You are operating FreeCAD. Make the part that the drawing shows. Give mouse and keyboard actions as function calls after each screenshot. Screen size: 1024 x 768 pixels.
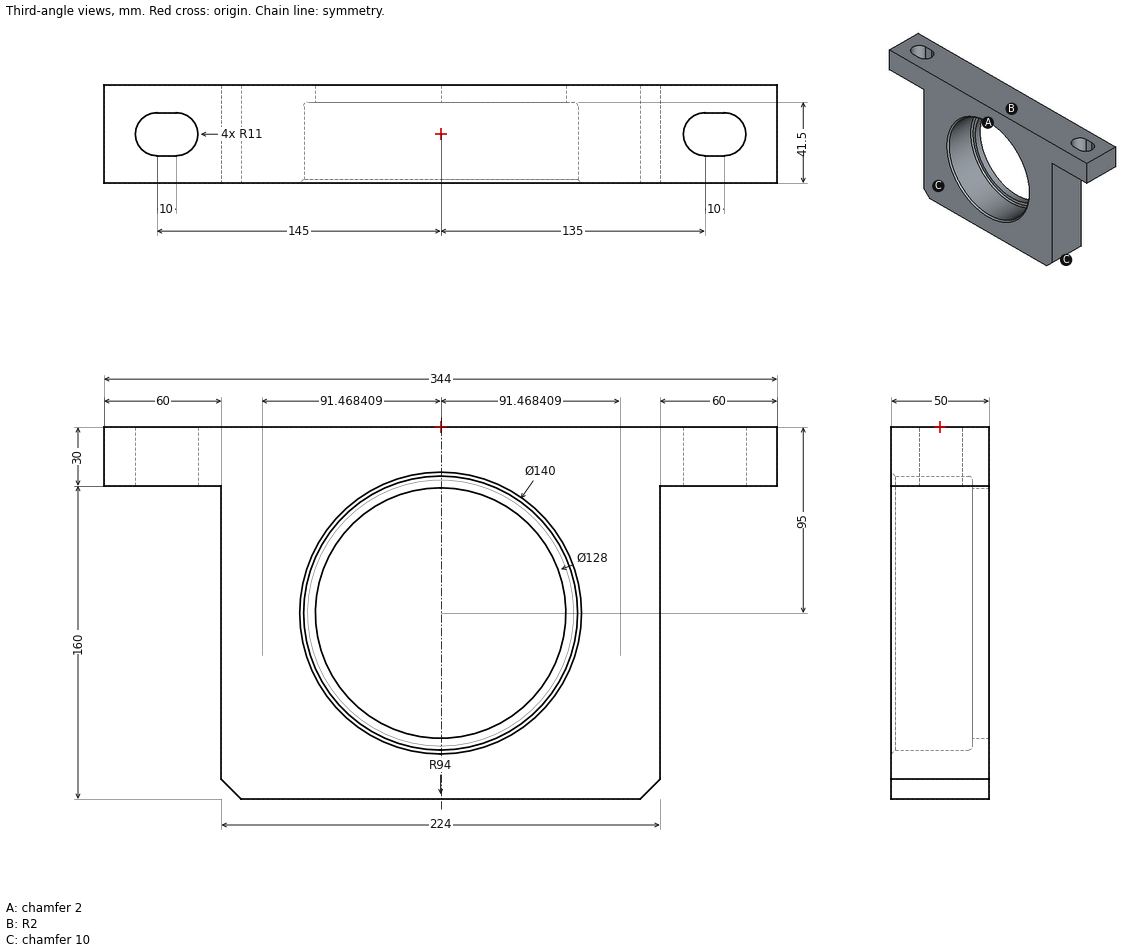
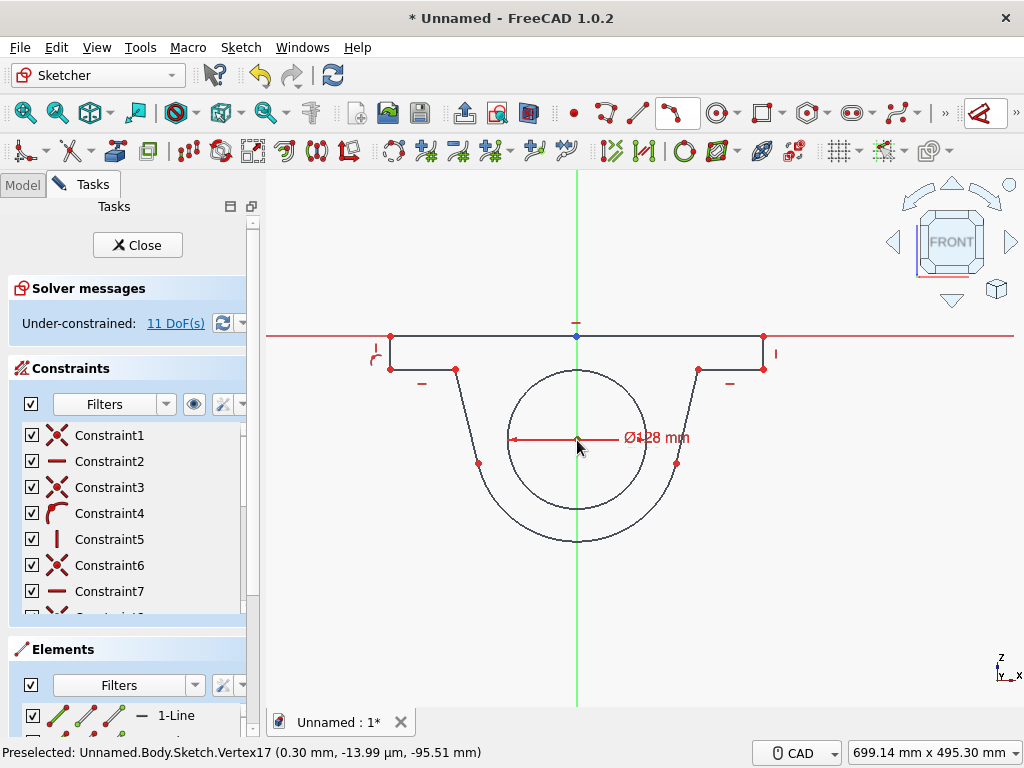
click(577, 645)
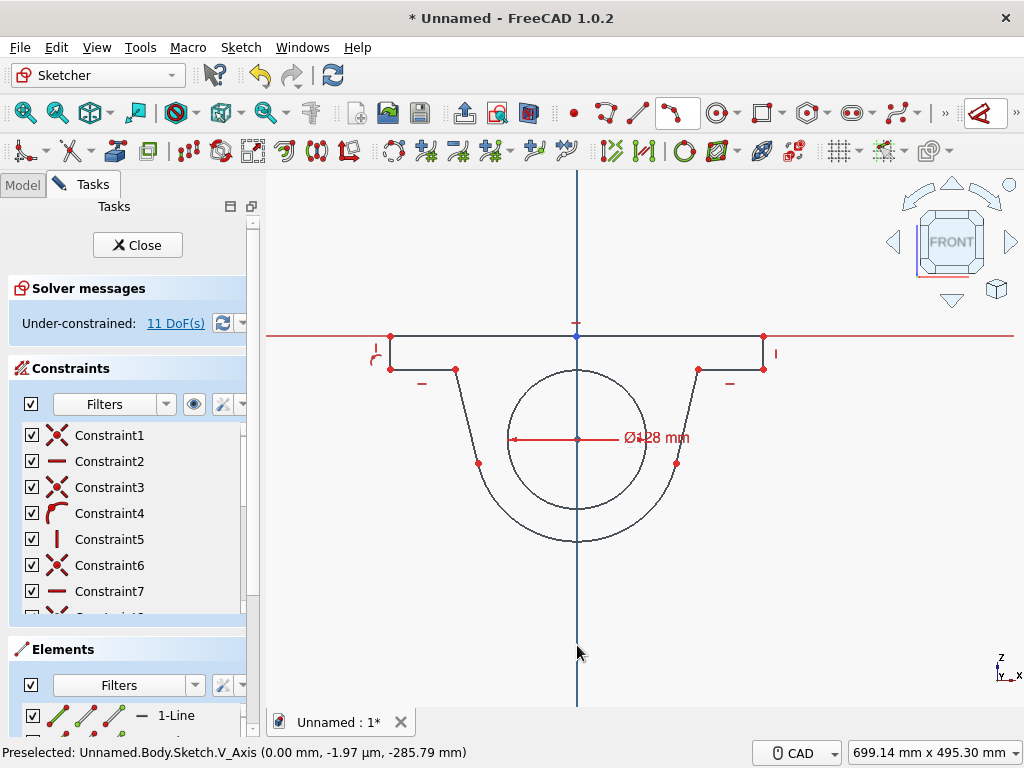
key(c)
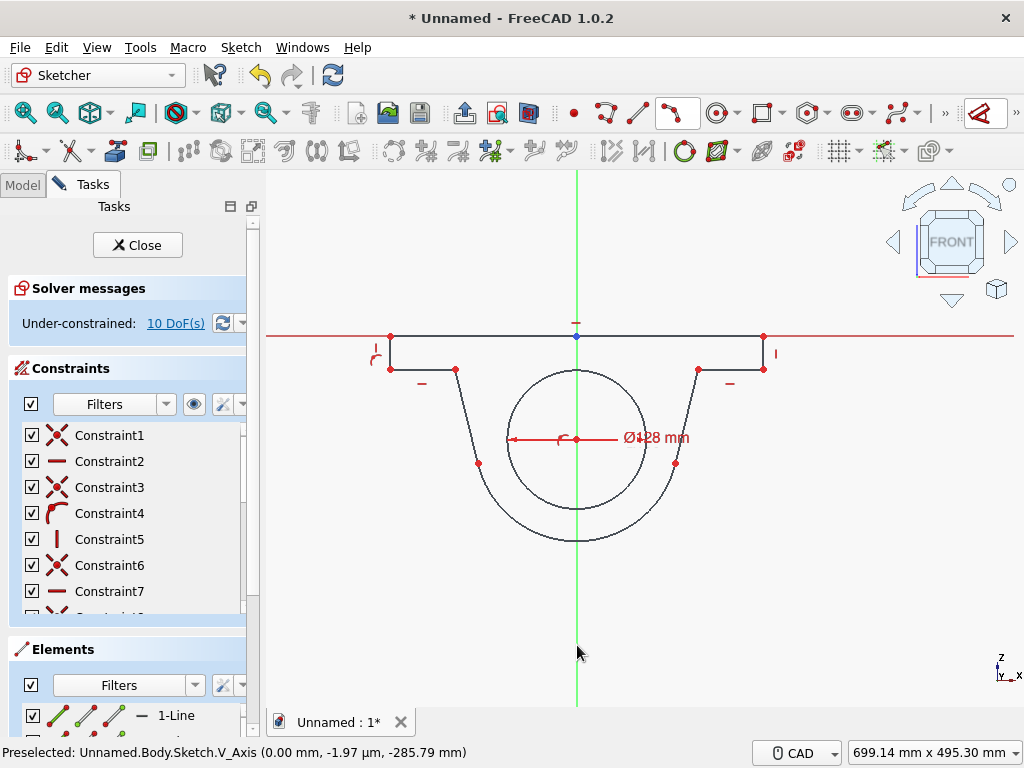
click(390, 370)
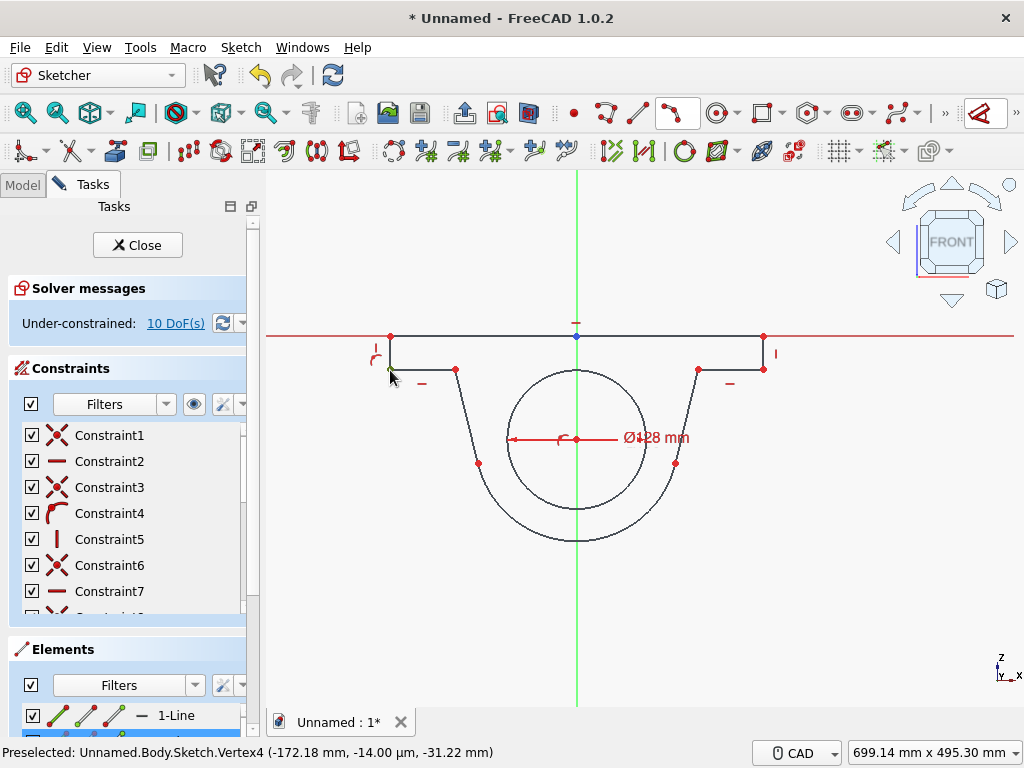
click(763, 370)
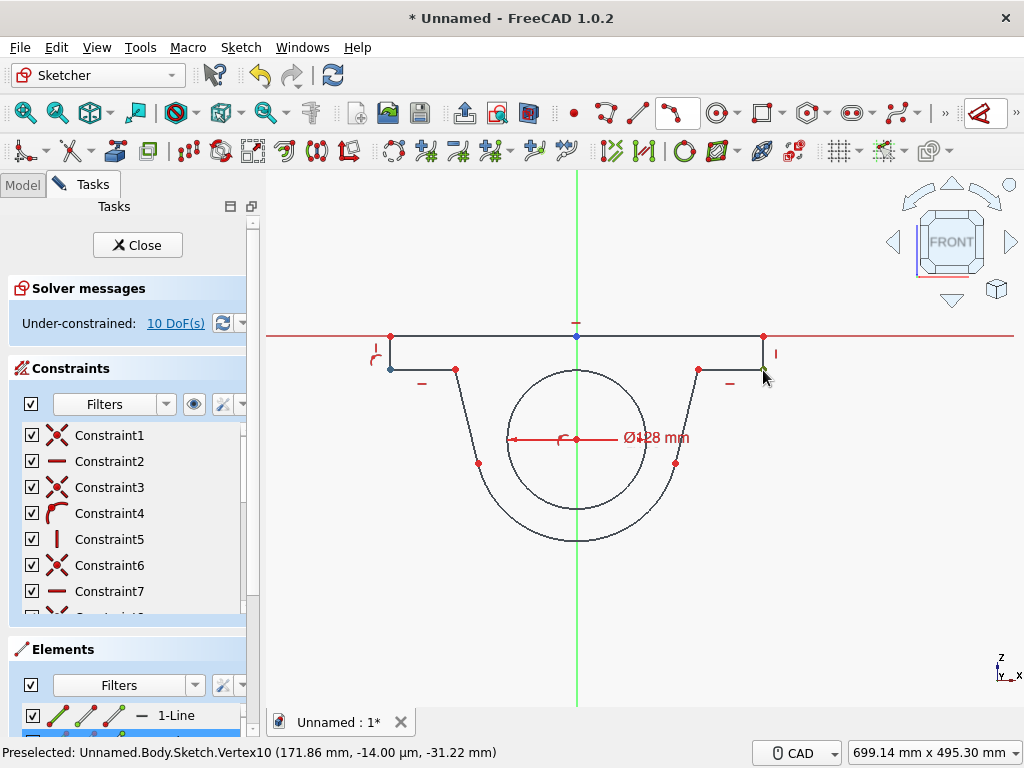
click(577, 645)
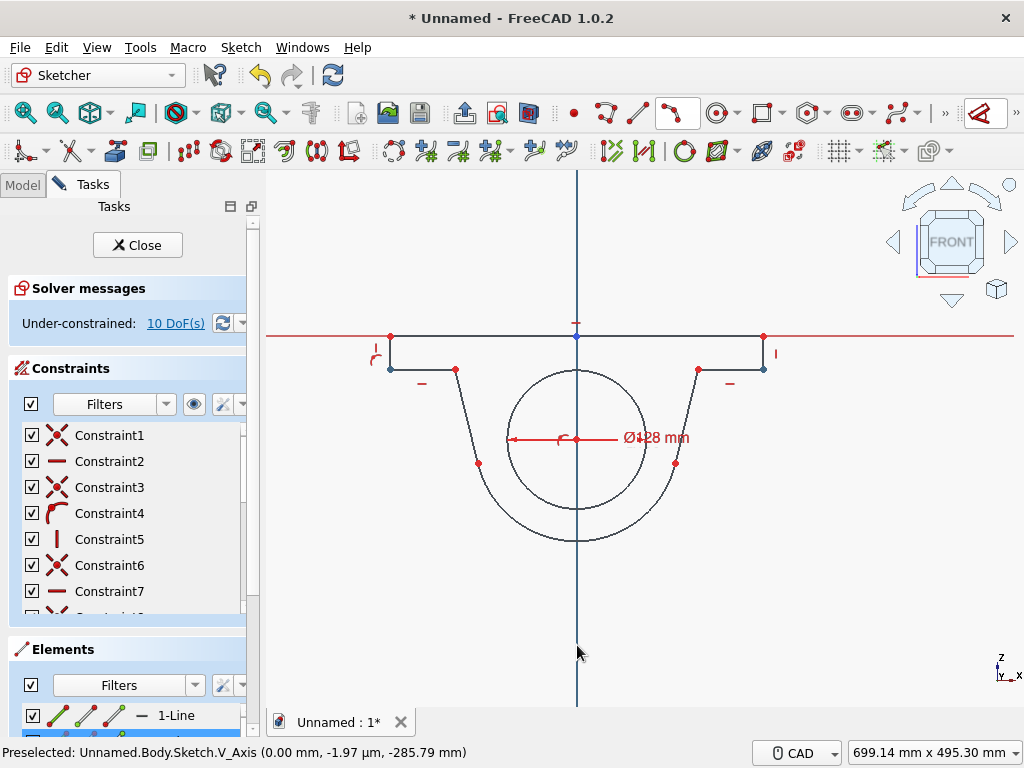
key(s)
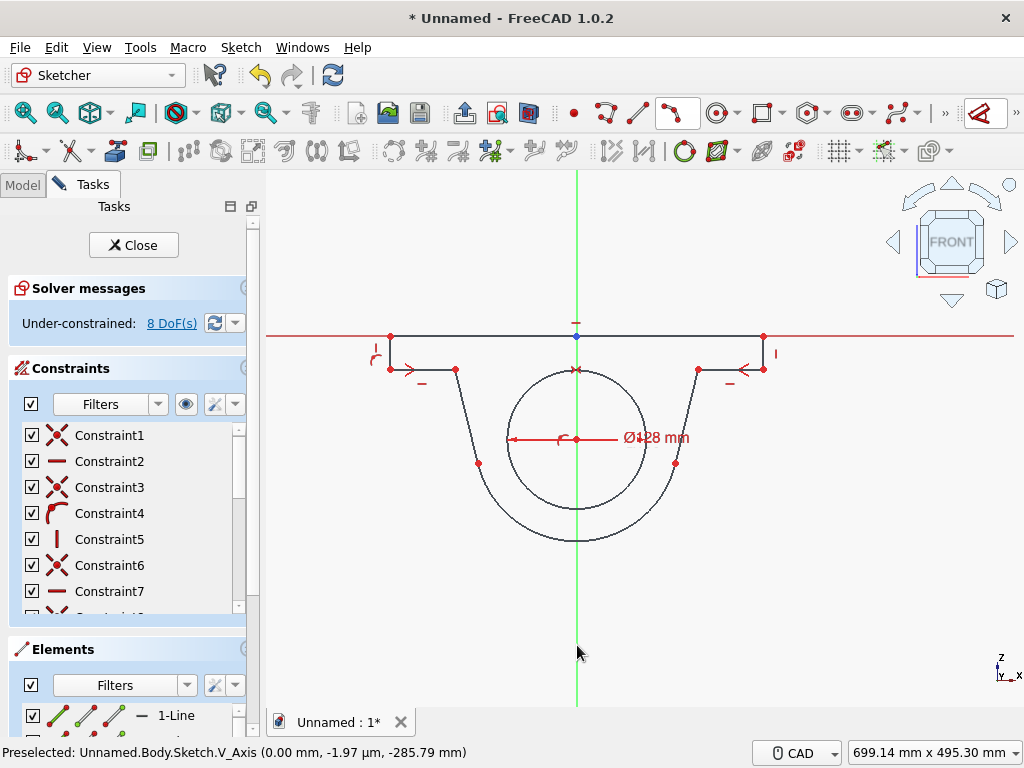
key(d)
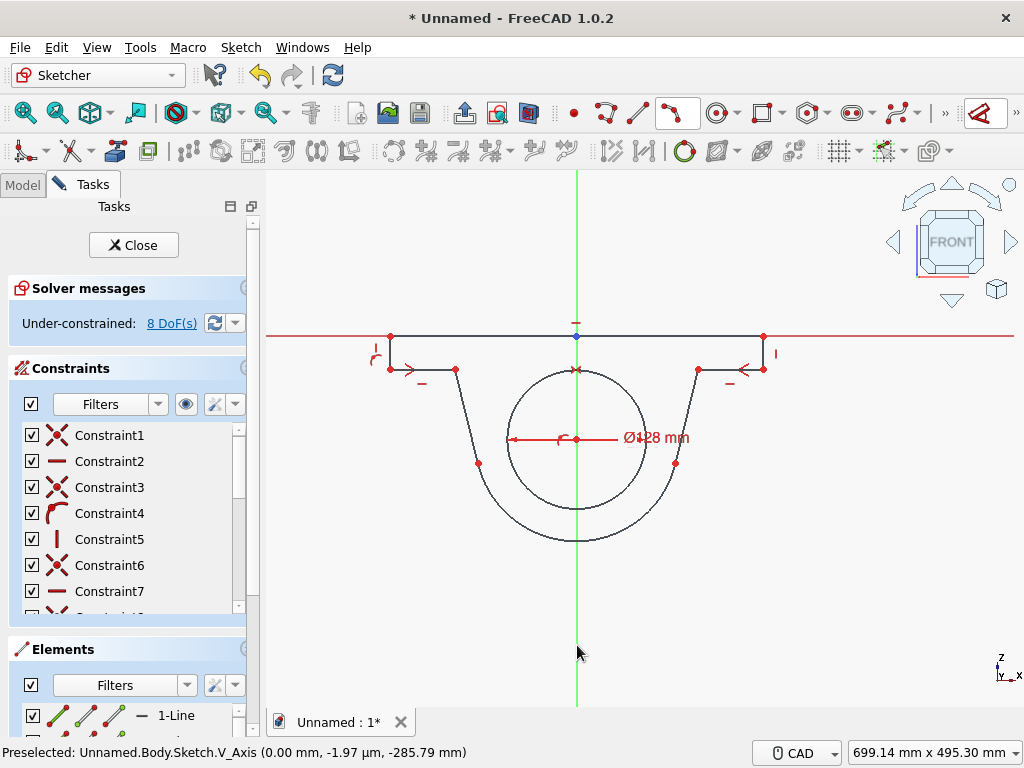
click(525, 527)
click(509, 555)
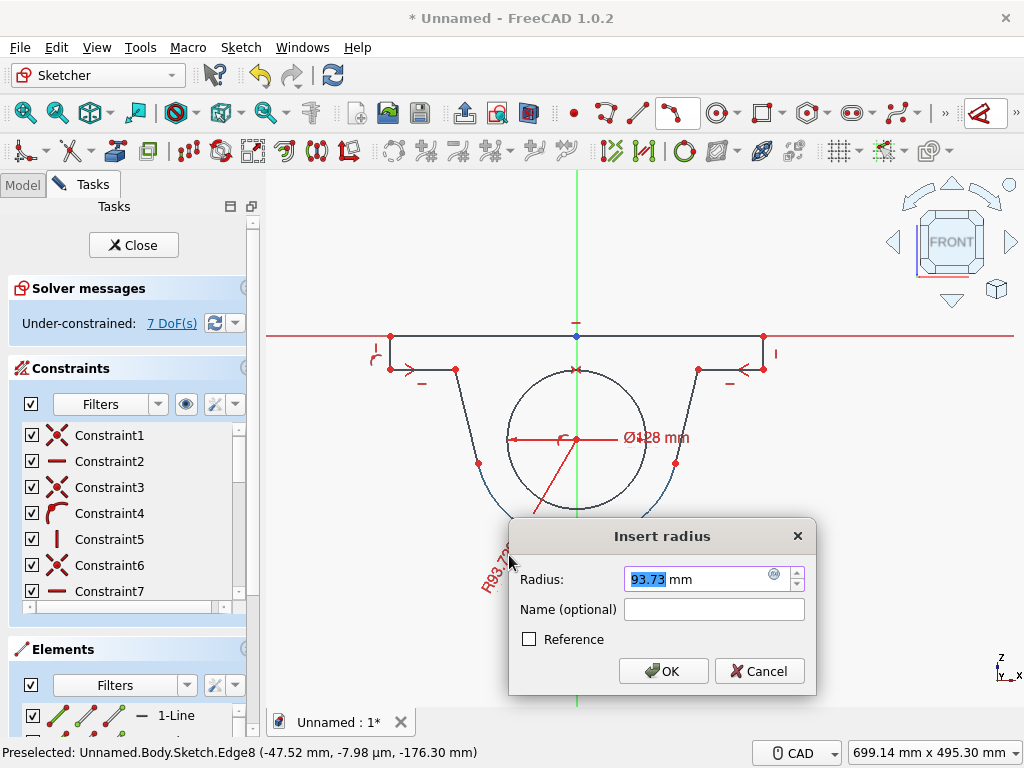
text(94)
key(Return)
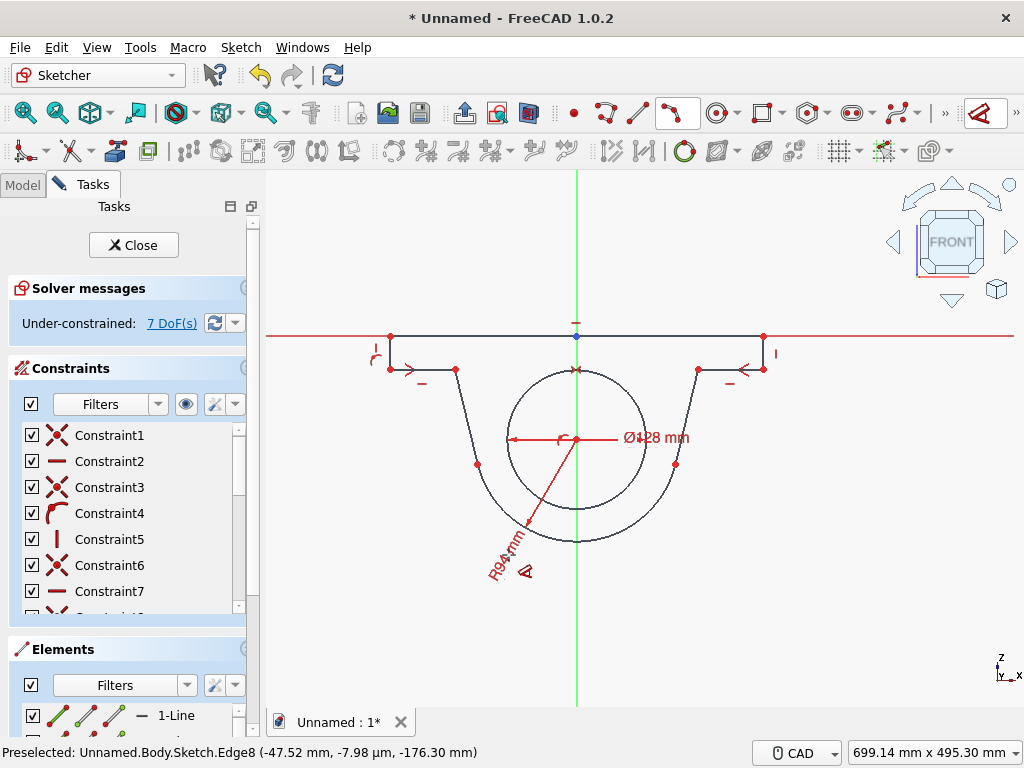
click(436, 370)
click(423, 404)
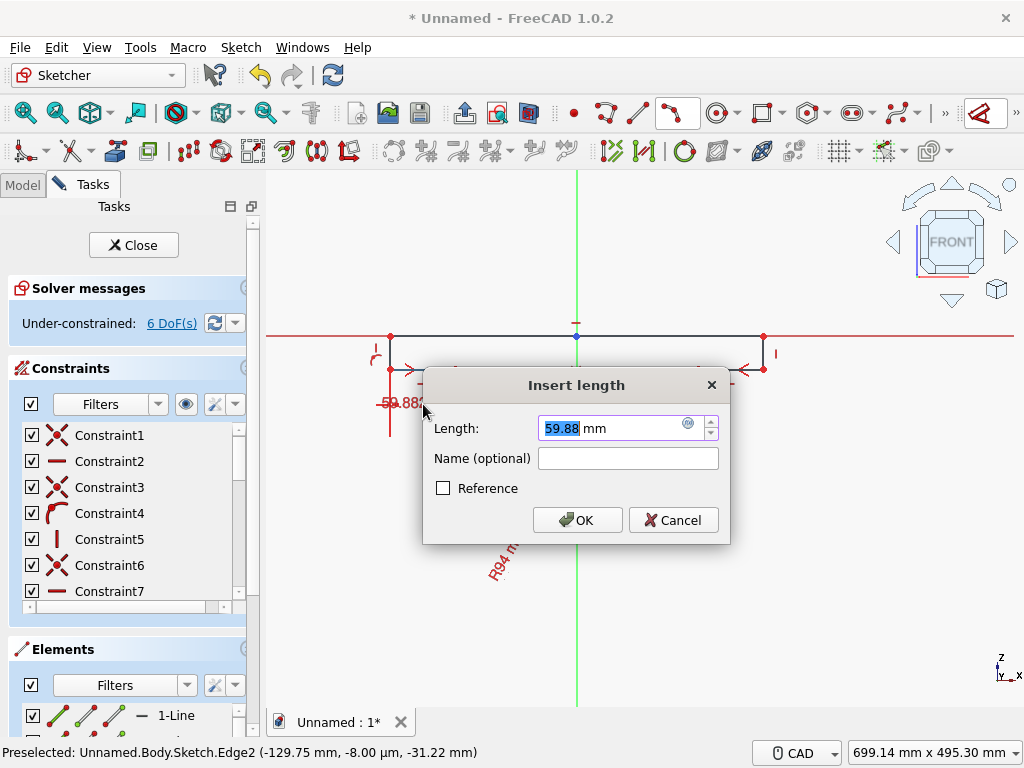
text(60)
key(Return)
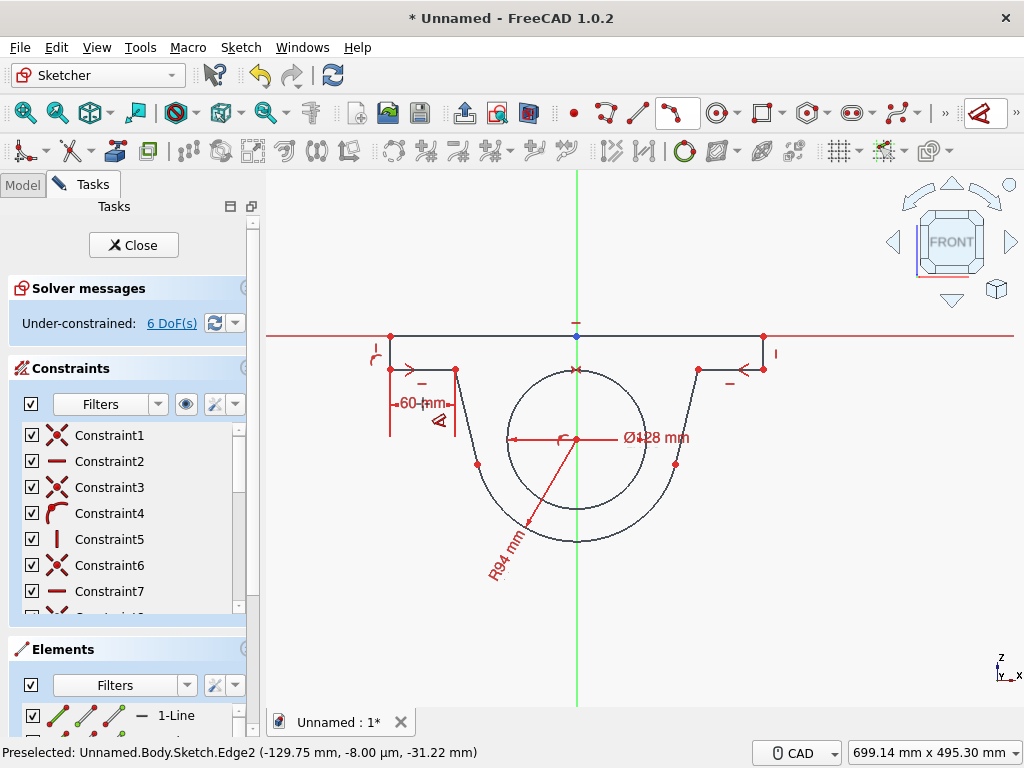
scroll(390, 360, up, 2)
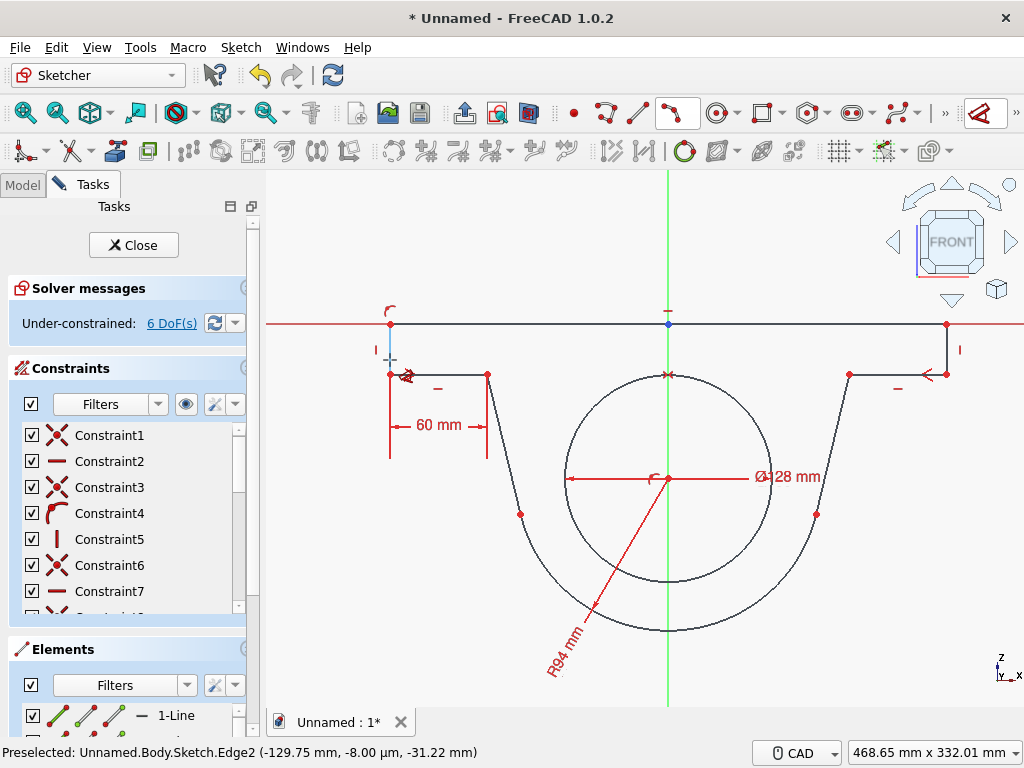
click(390, 360)
click(356, 349)